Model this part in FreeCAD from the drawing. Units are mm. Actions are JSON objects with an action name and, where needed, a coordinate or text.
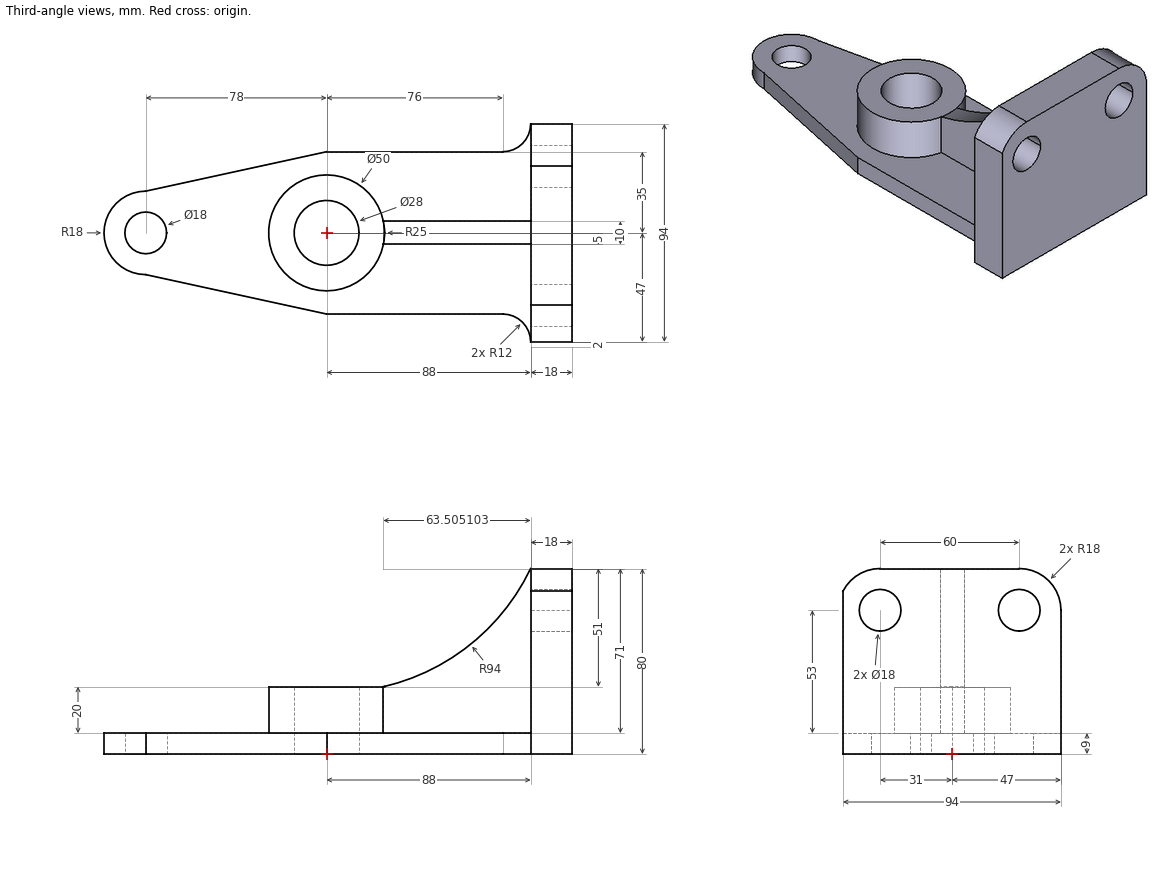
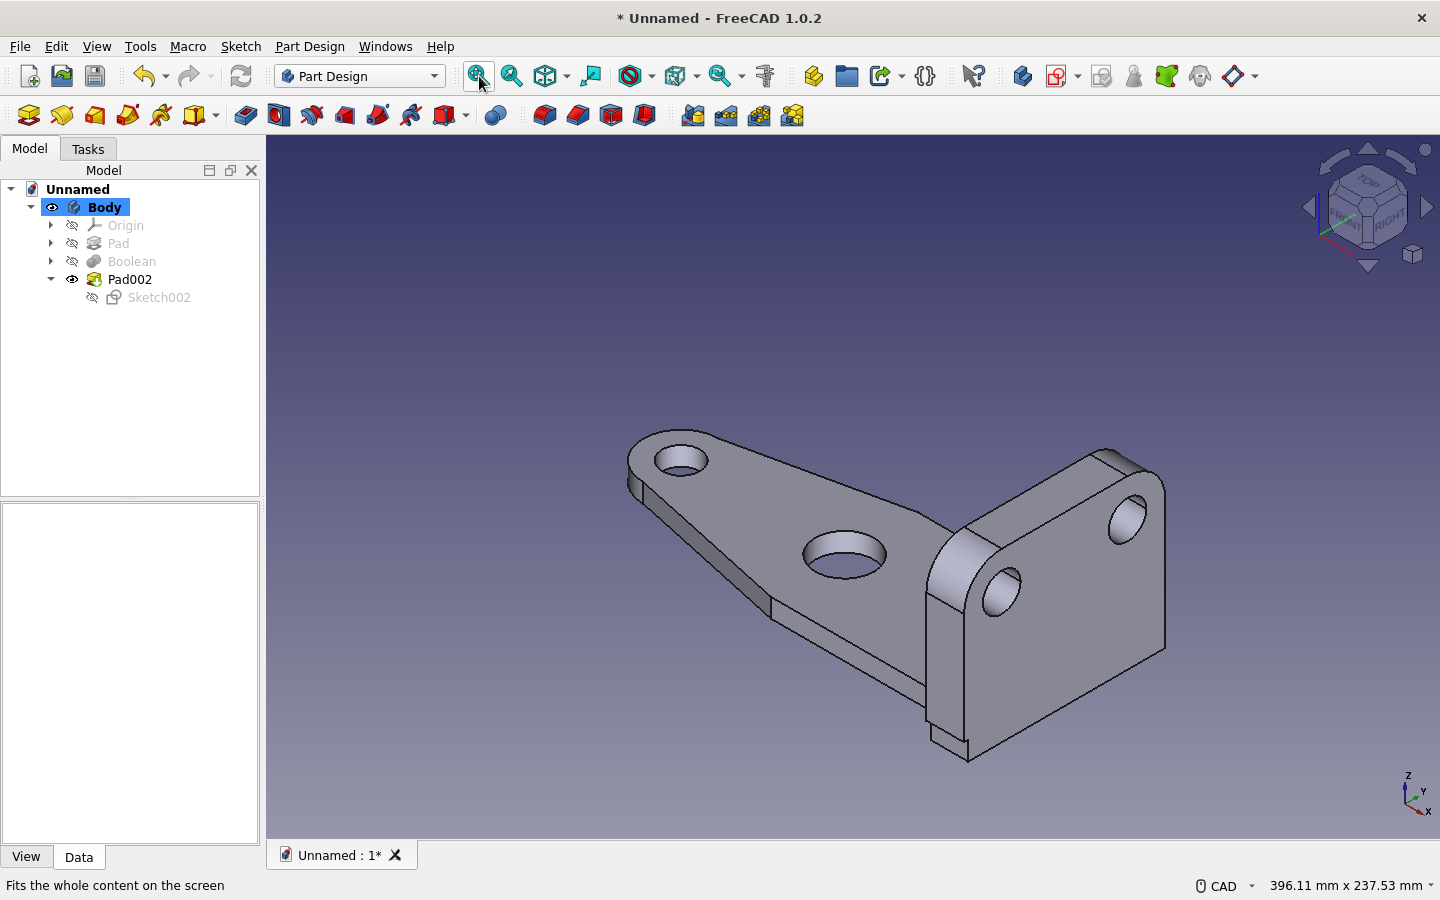
{"action": "left_click", "coordinate": [918, 629]}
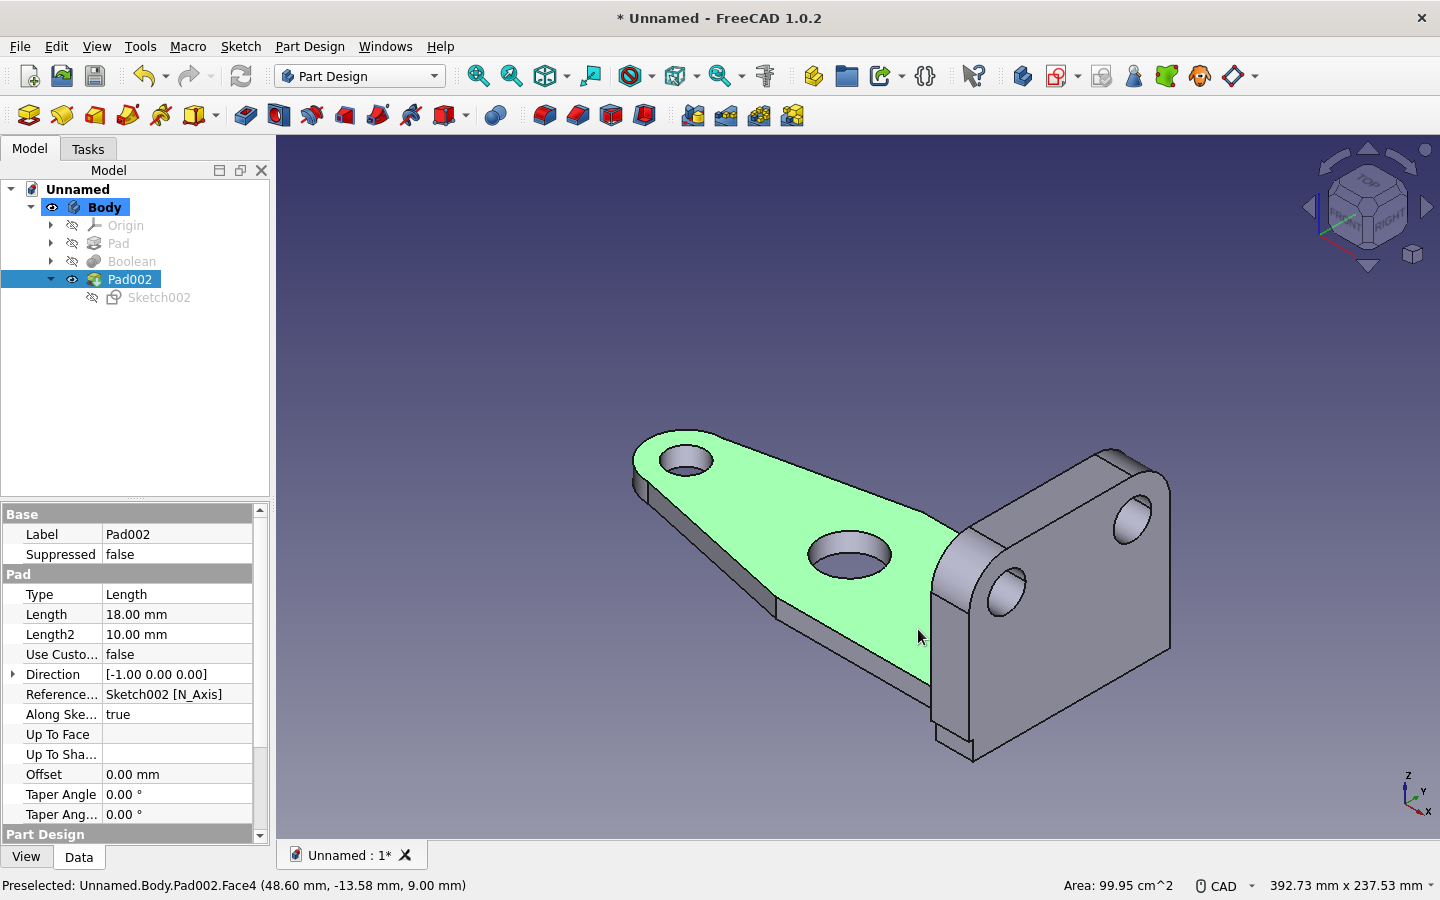
{"action": "left_click", "coordinate": [1056, 76]}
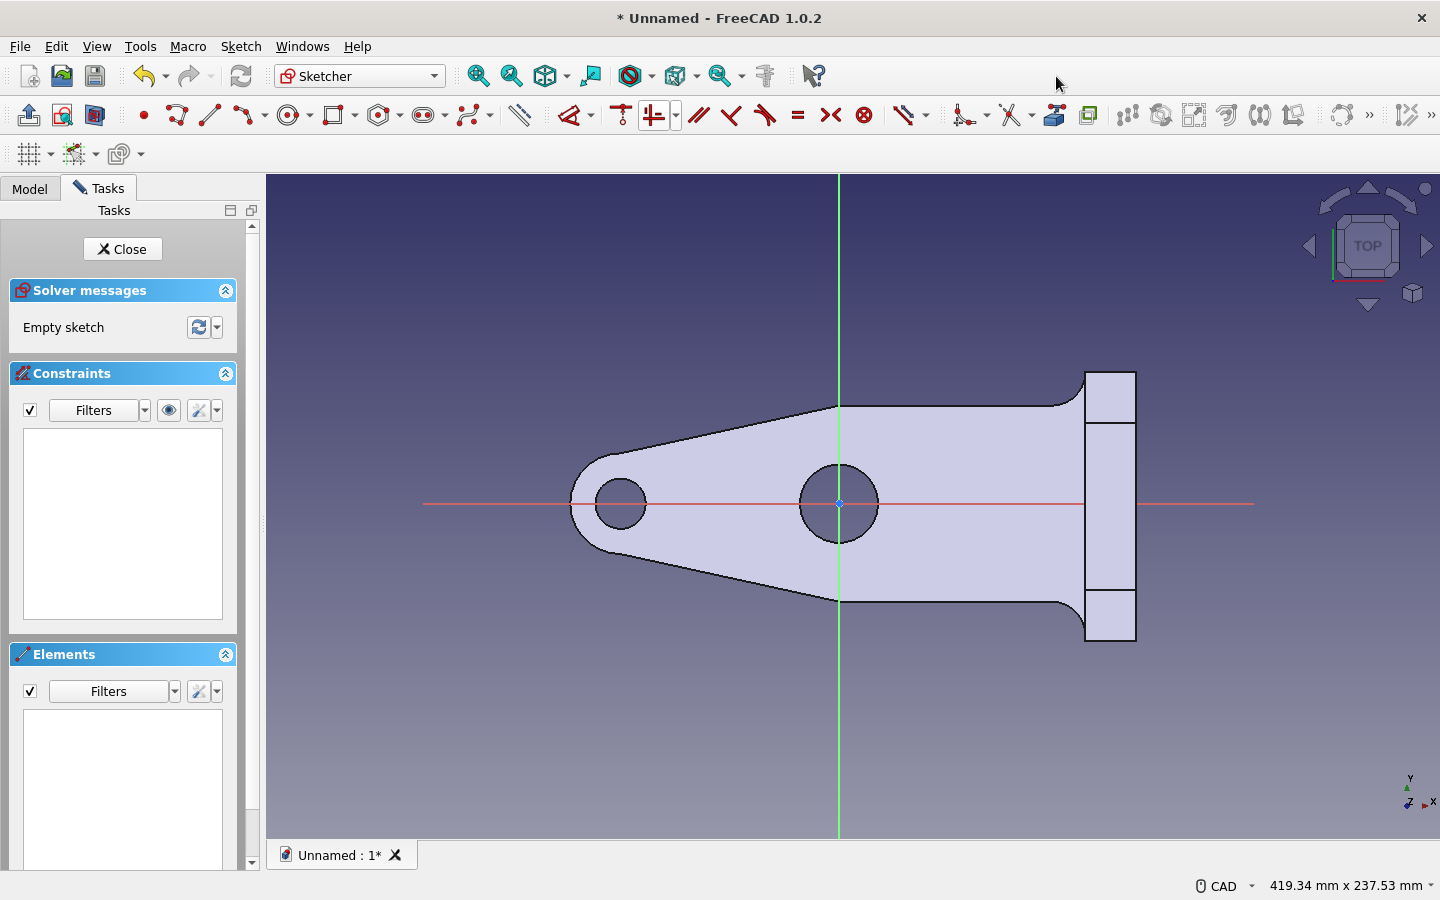
{"action": "scroll", "coordinate": [862, 502], "scroll_direction": "up", "scroll_amount": 6}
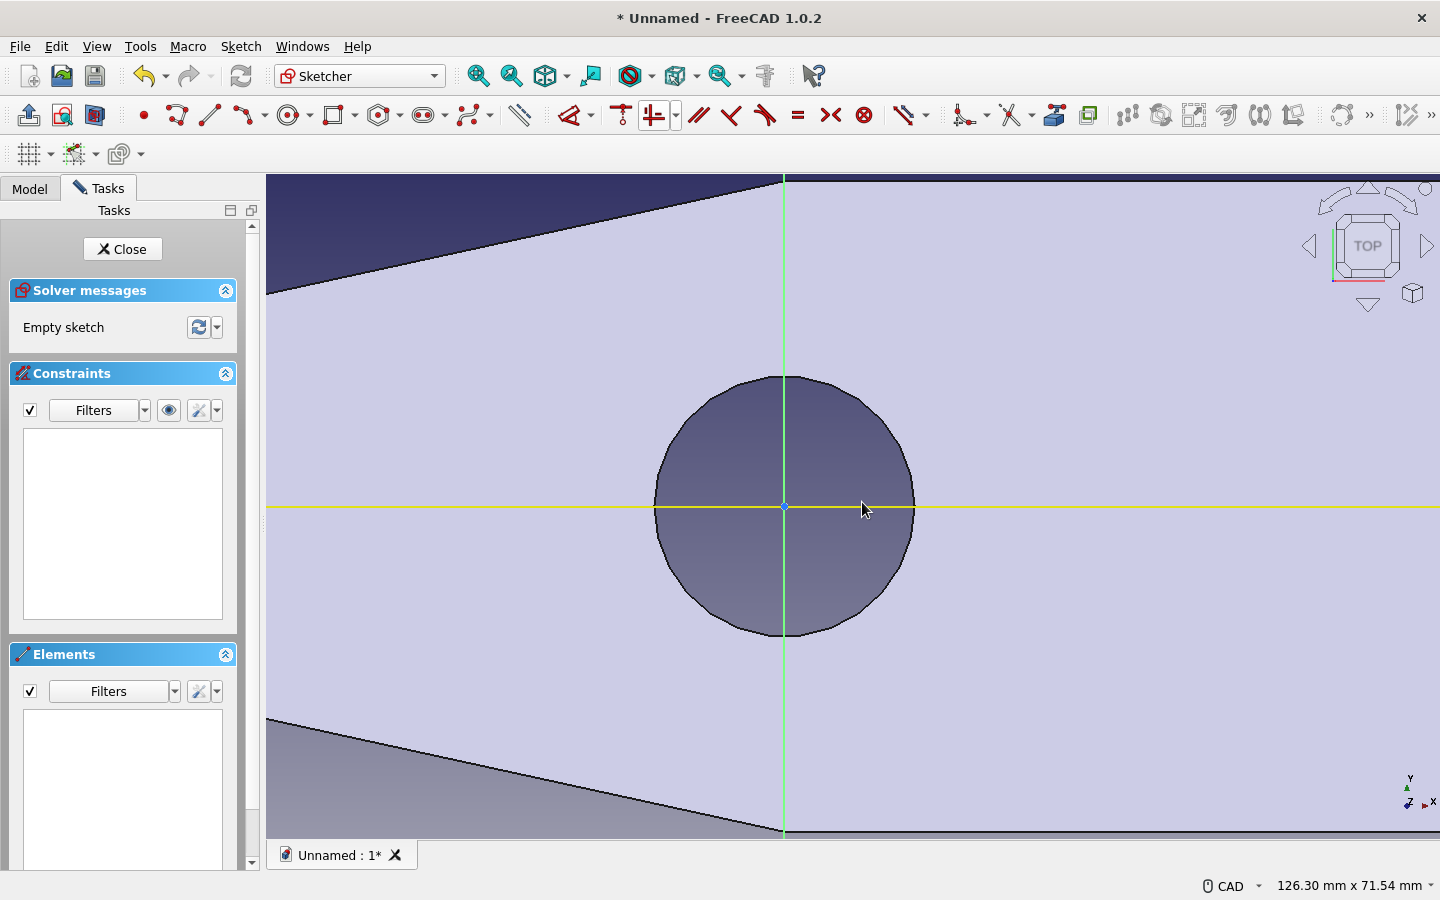
{"action": "key", "text": "g c"}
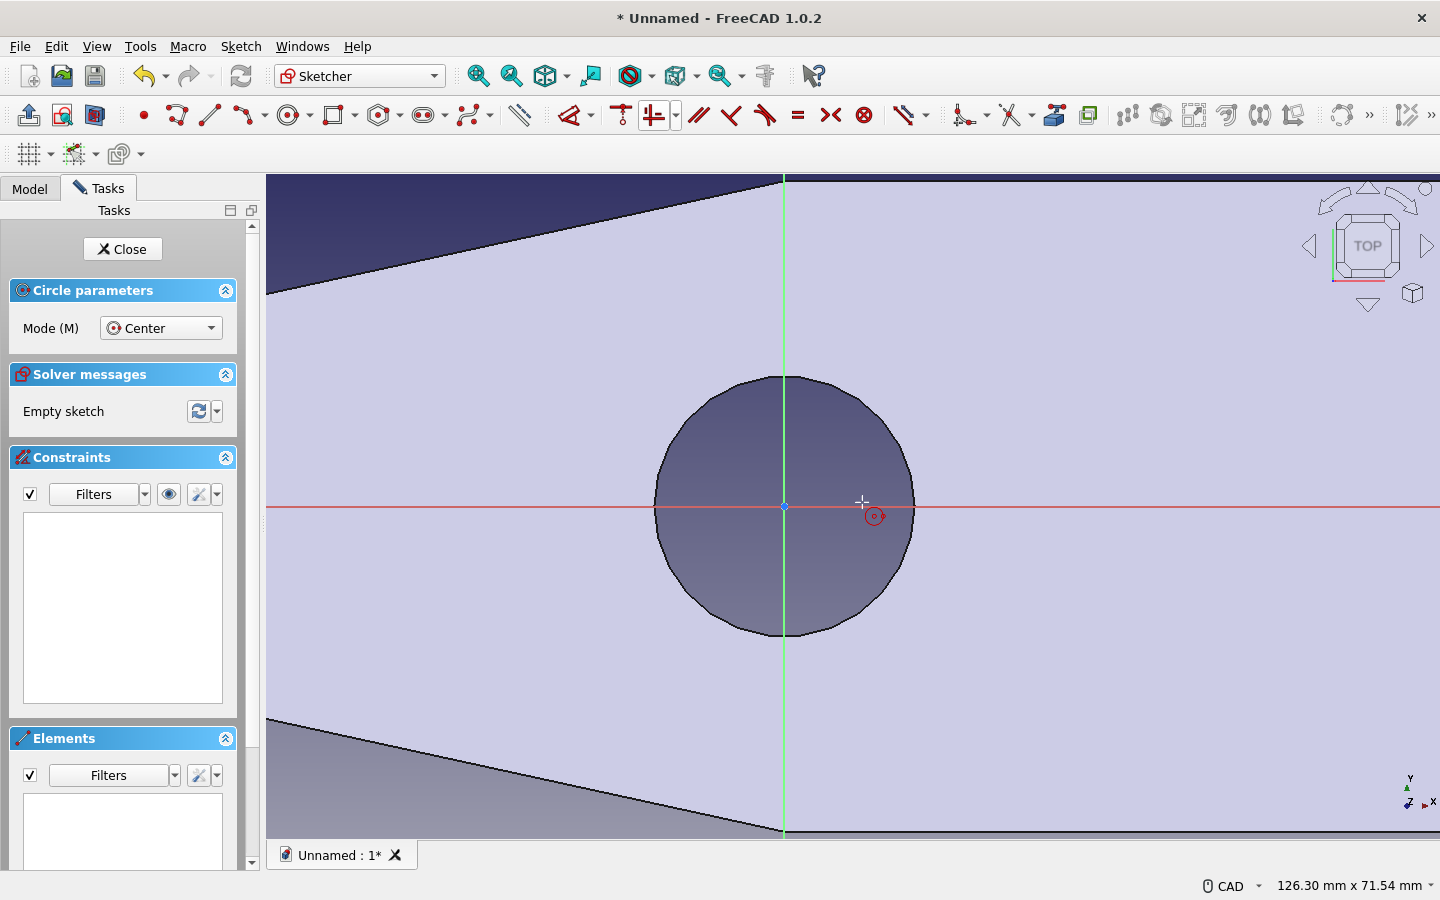
{"action": "left_click", "coordinate": [784, 506]}
{"action": "left_click", "coordinate": [949, 342]}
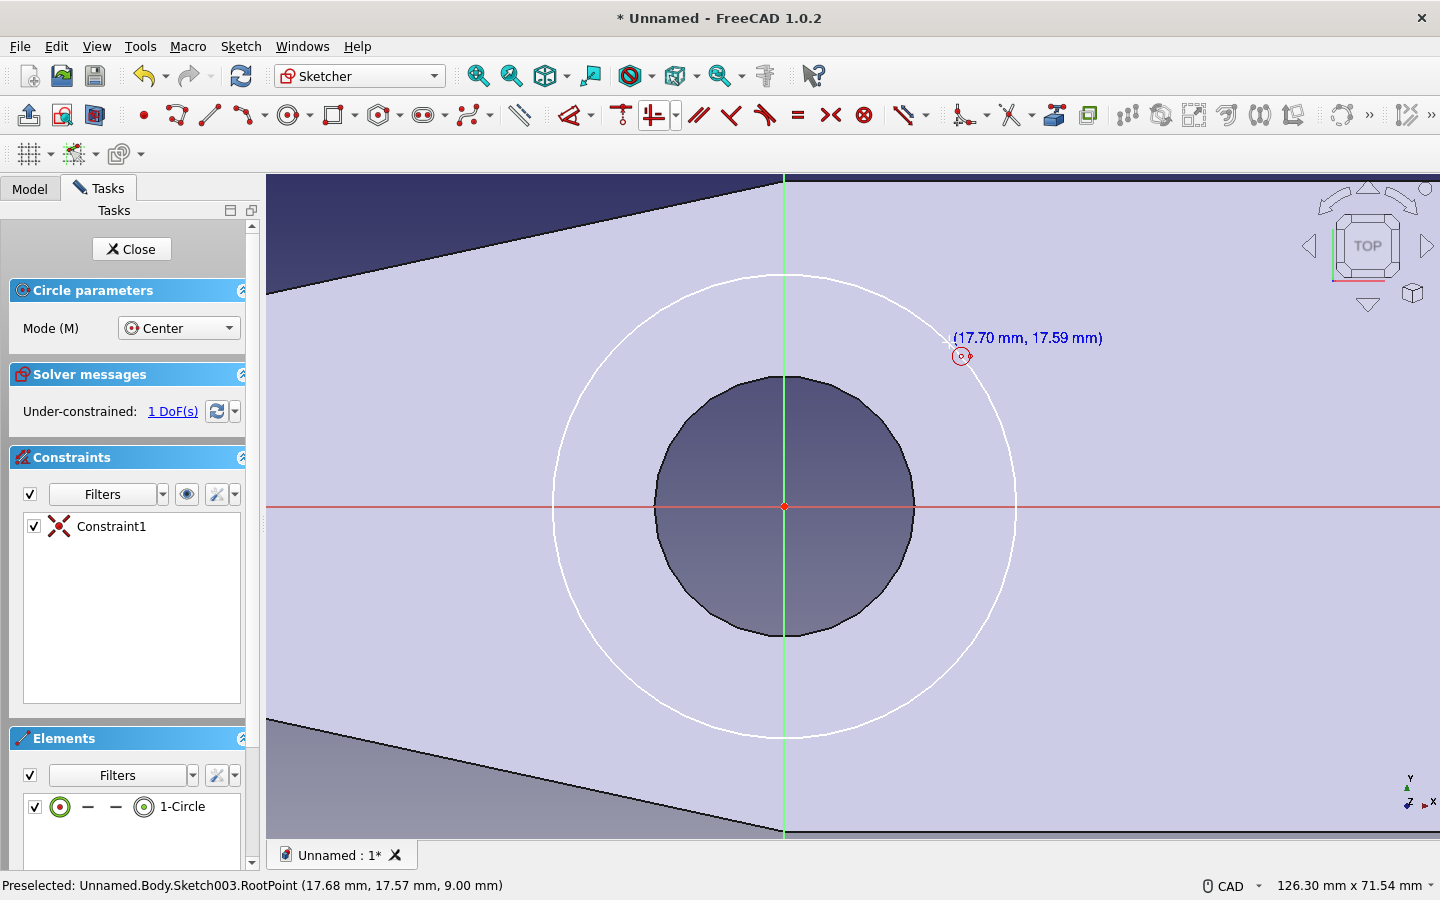
{"action": "left_click", "coordinate": [784, 506]}
{"action": "left_click", "coordinate": [876, 414]}
{"action": "key", "text": "Escape"}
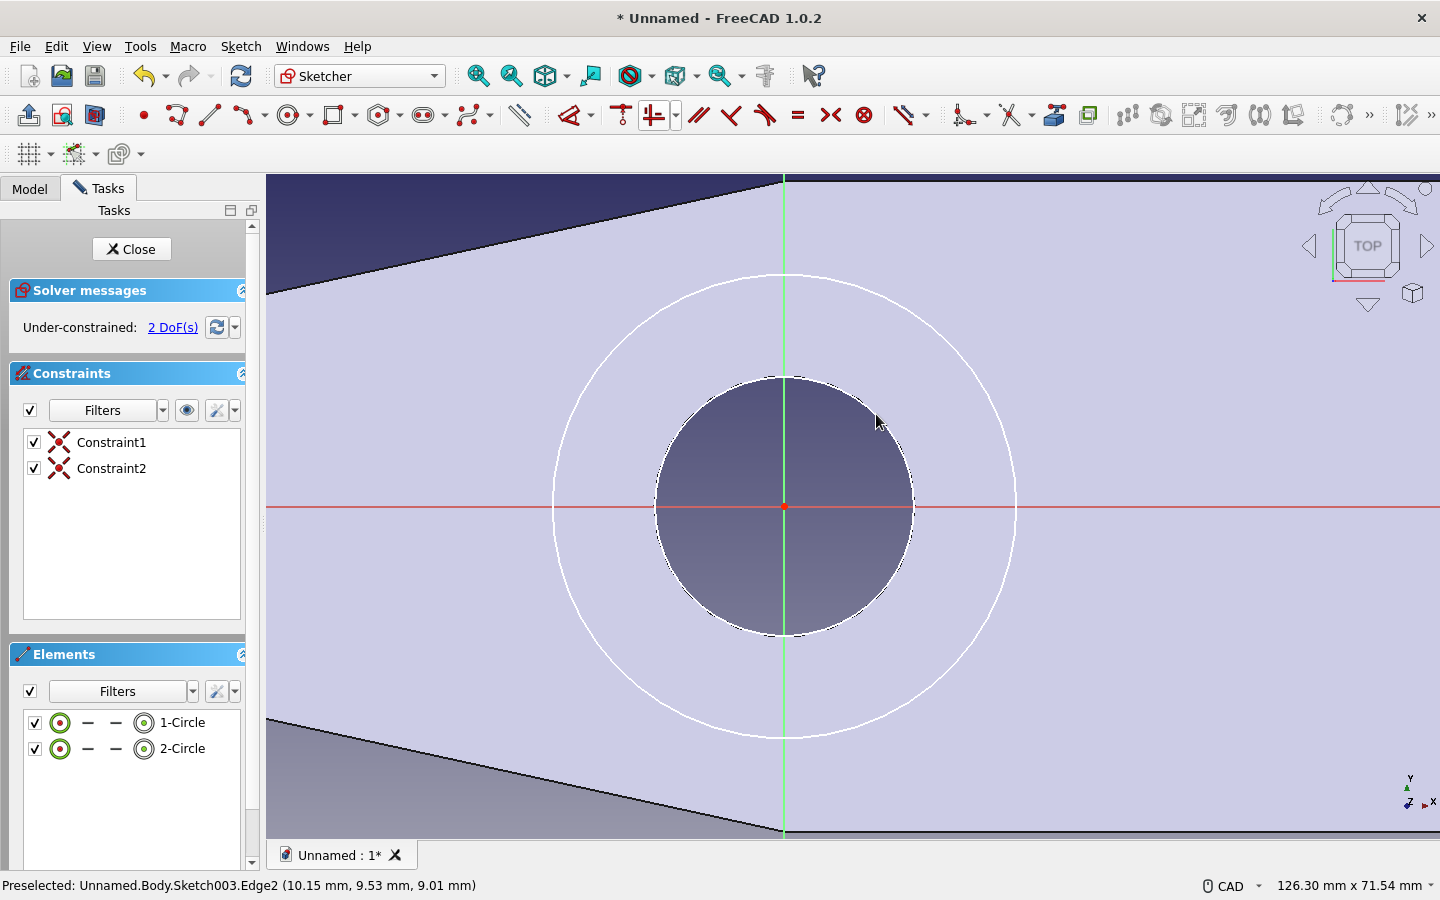
{"action": "left_click", "coordinate": [568, 116]}